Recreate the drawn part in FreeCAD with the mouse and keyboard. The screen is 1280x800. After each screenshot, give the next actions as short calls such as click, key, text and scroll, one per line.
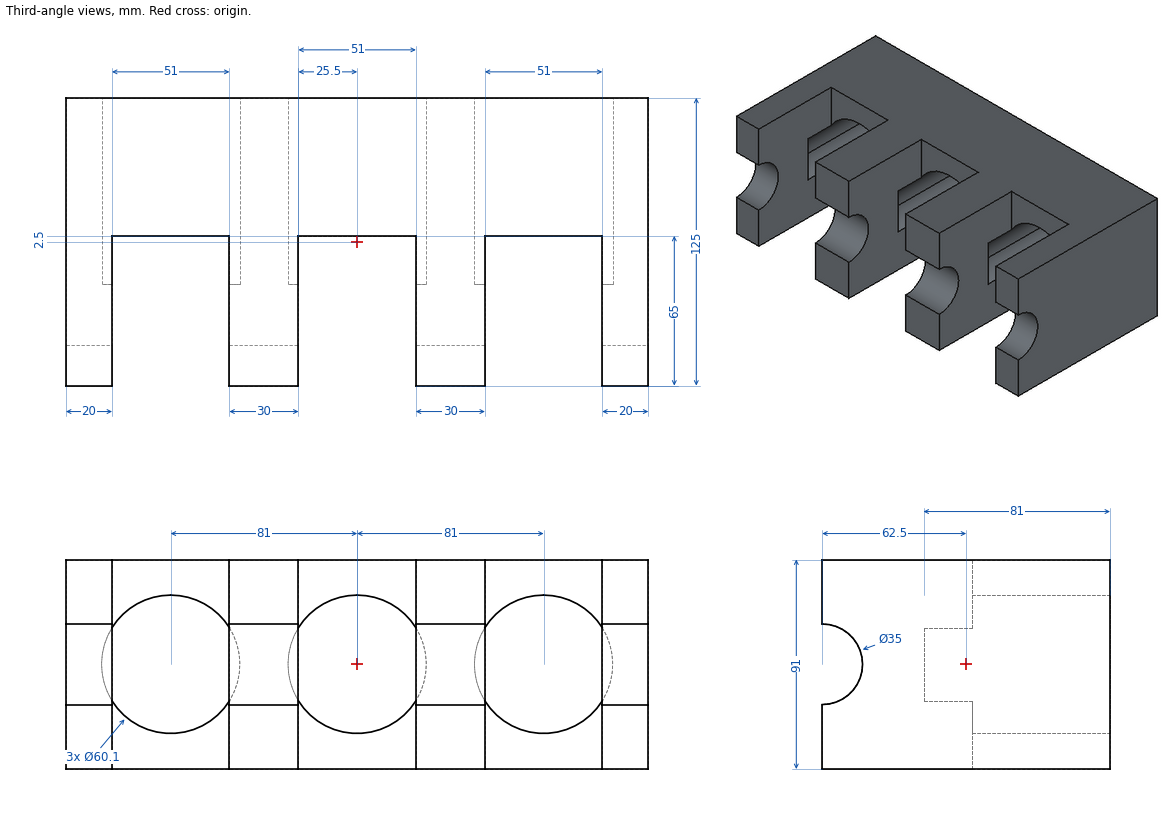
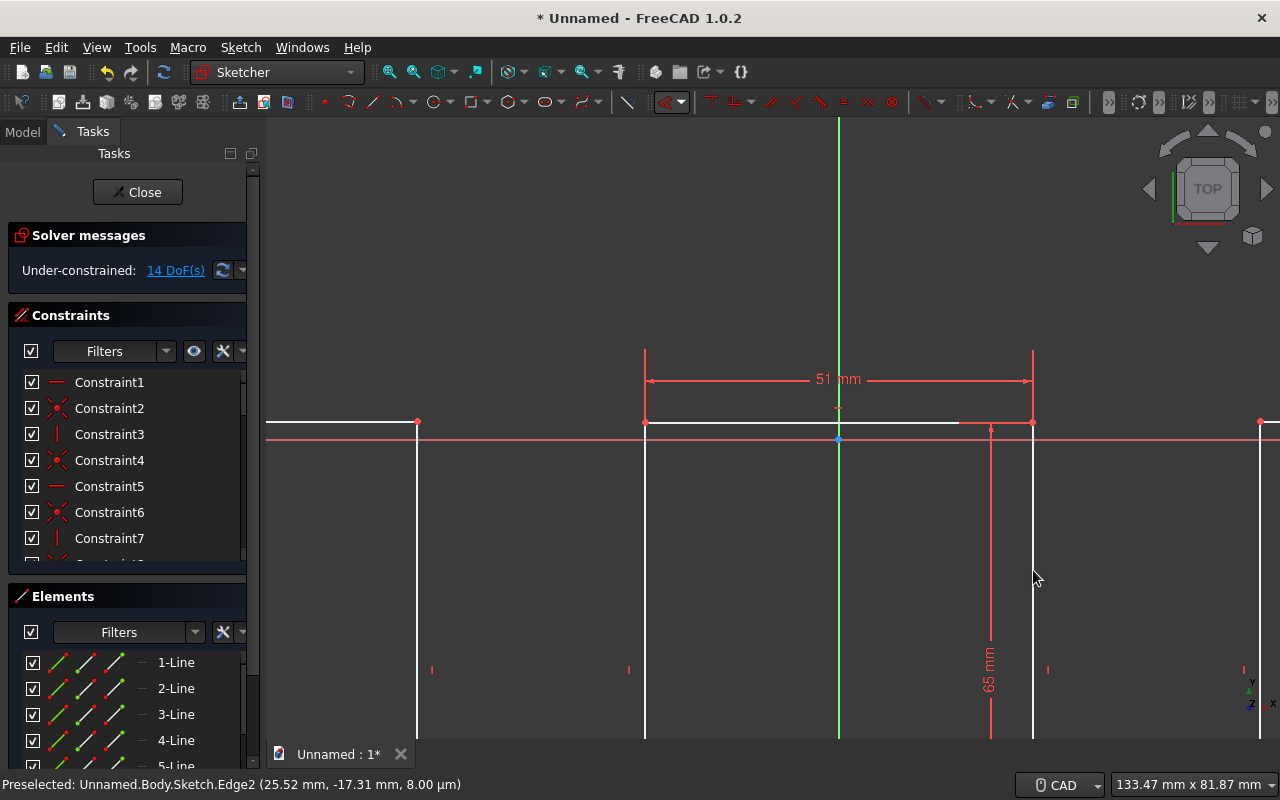
scroll(647, 423, down, 6)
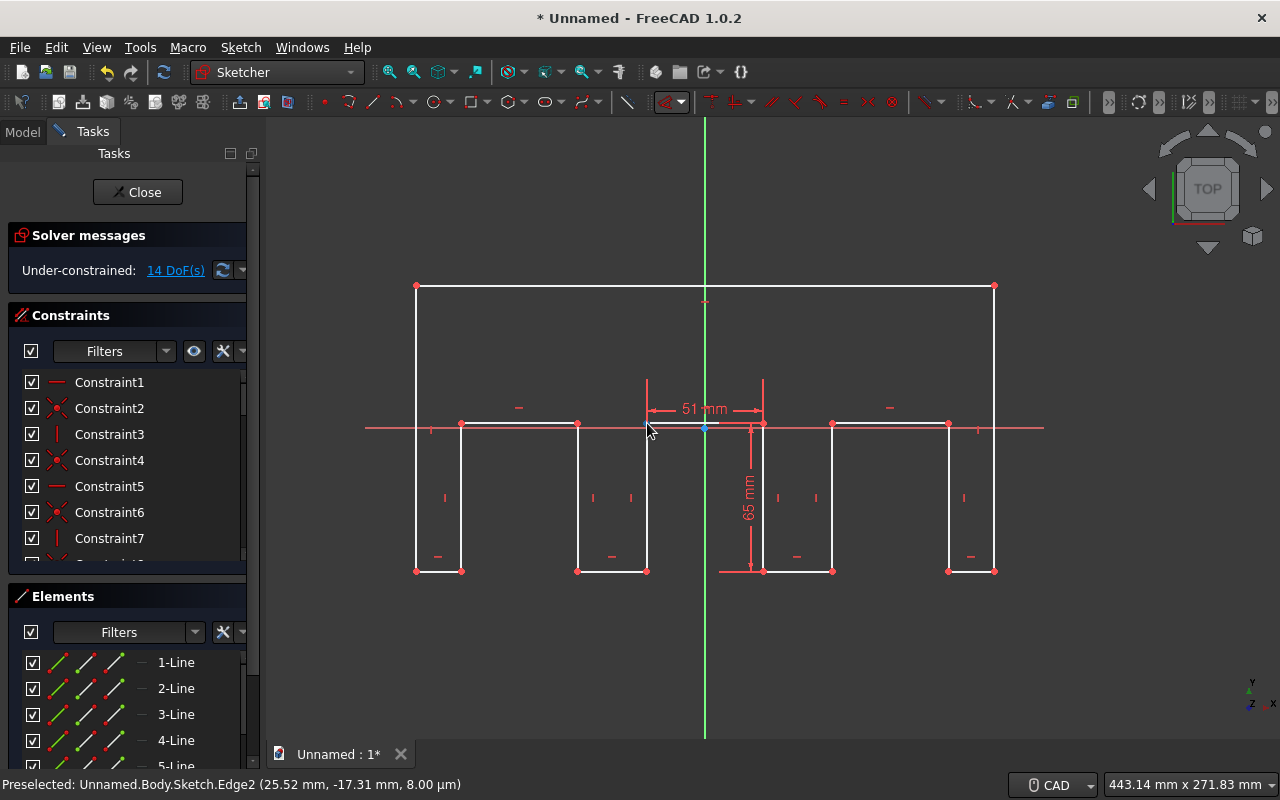
click(784, 572)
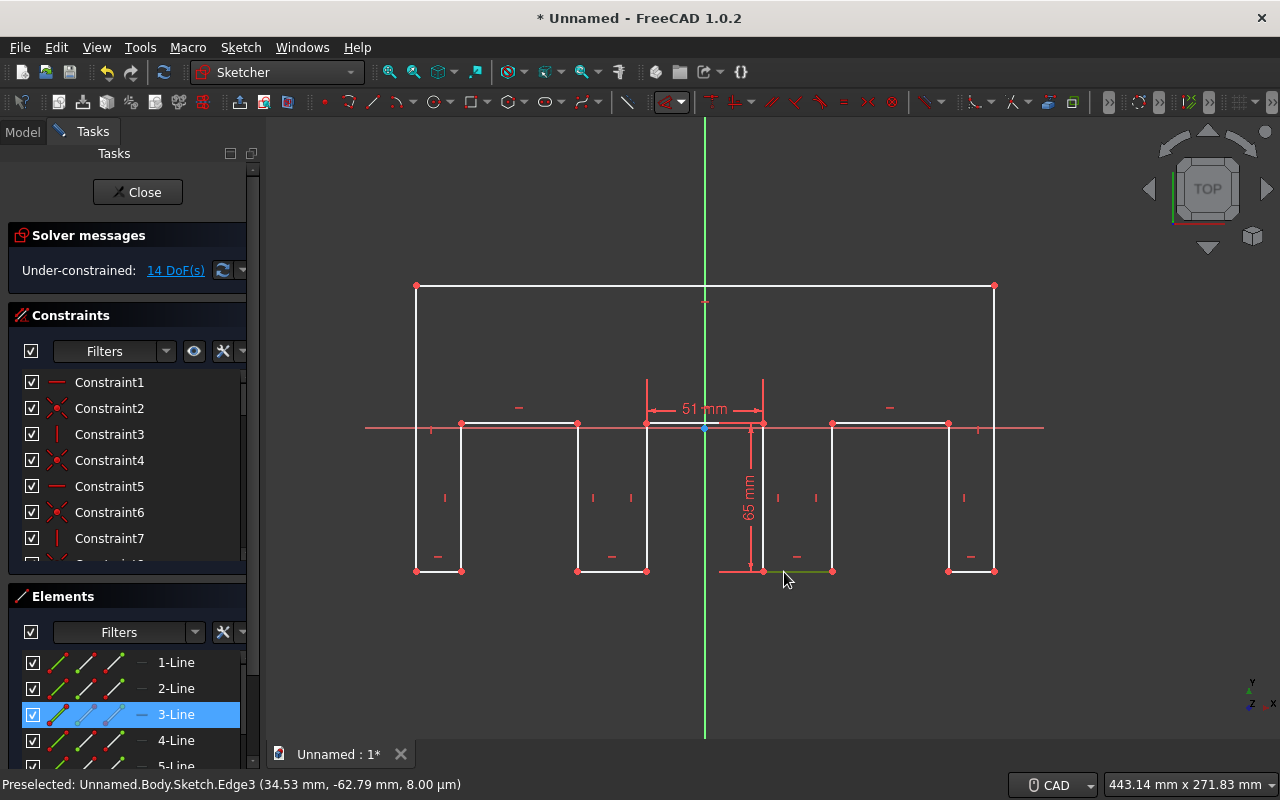
click(684, 102)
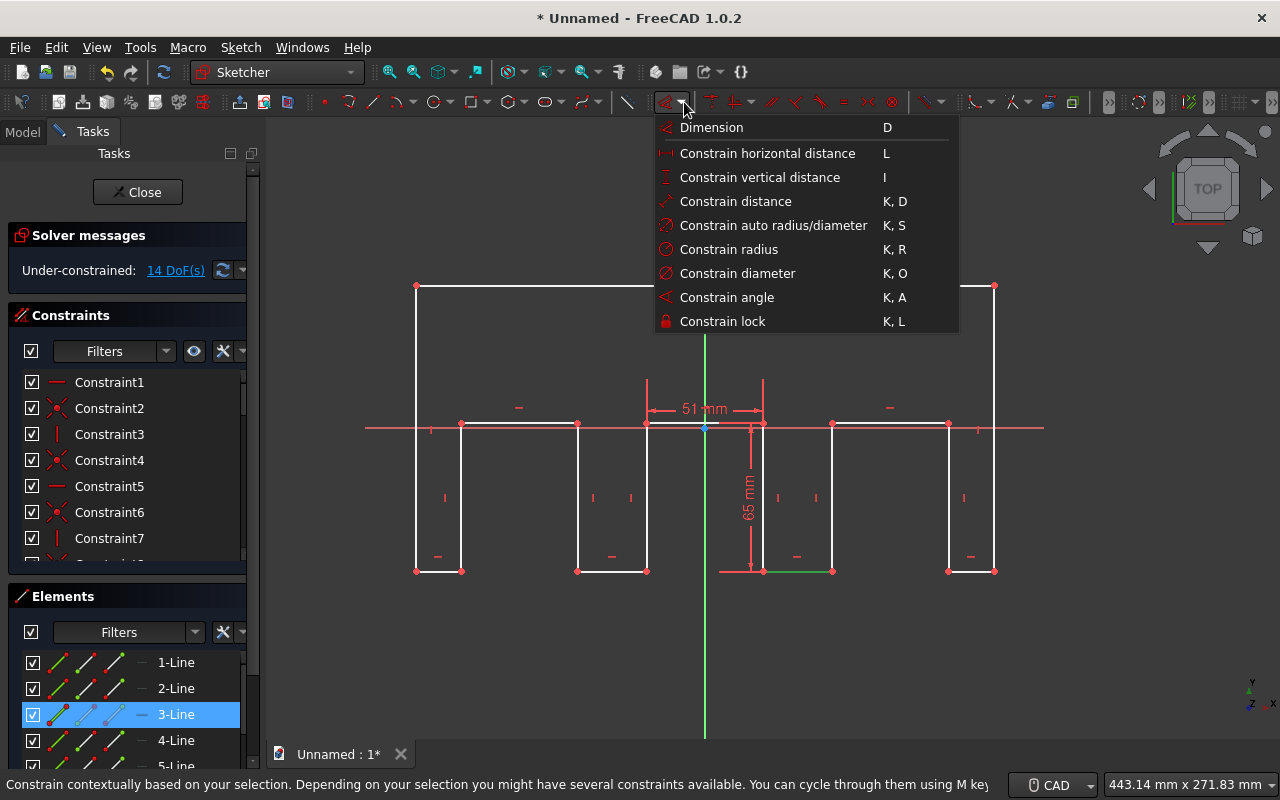
click(807, 153)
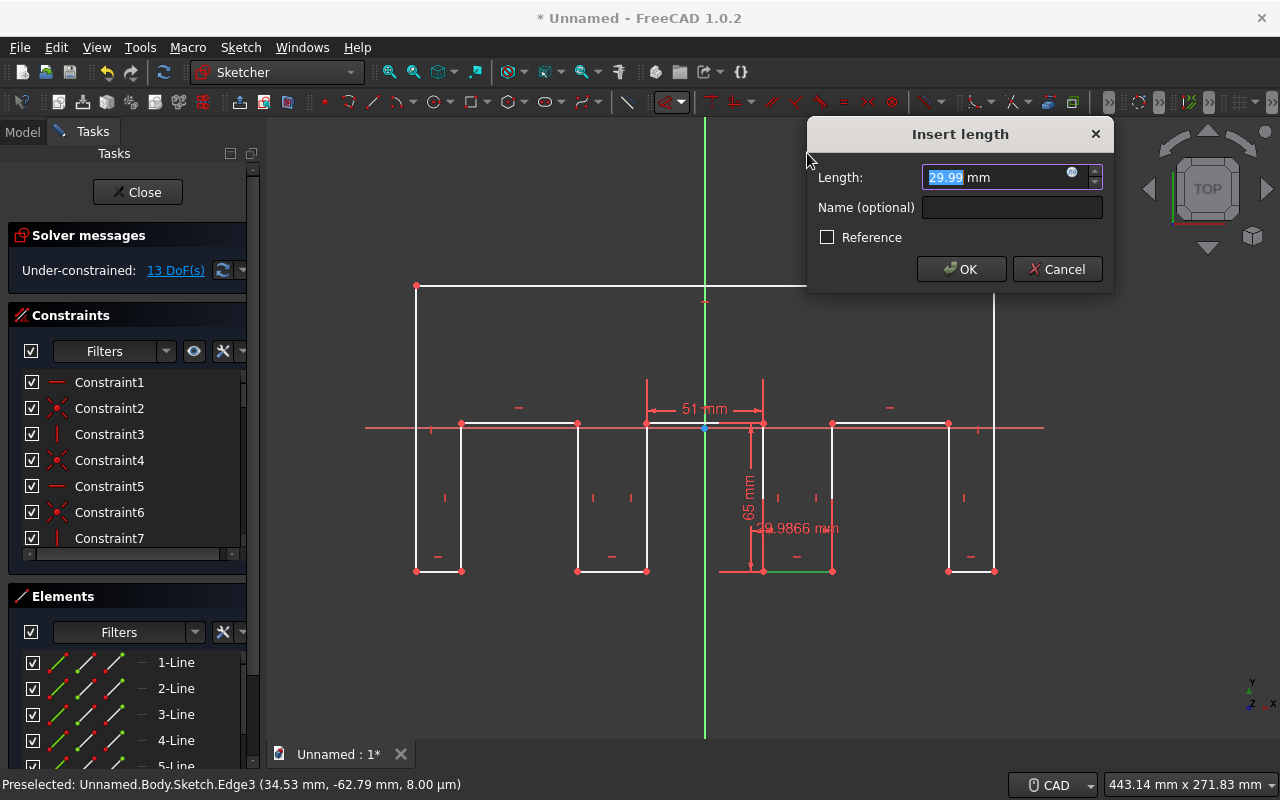
text(30)
key(Return)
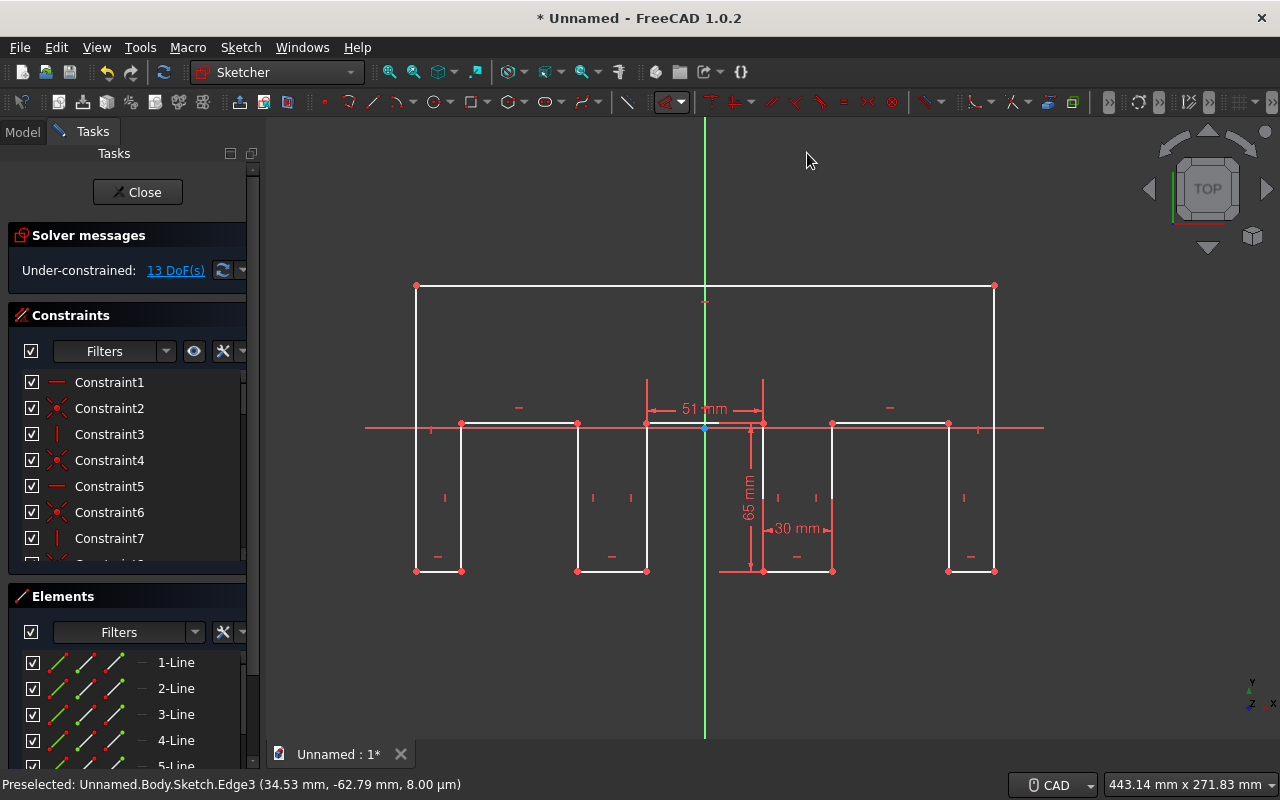
click(832, 527)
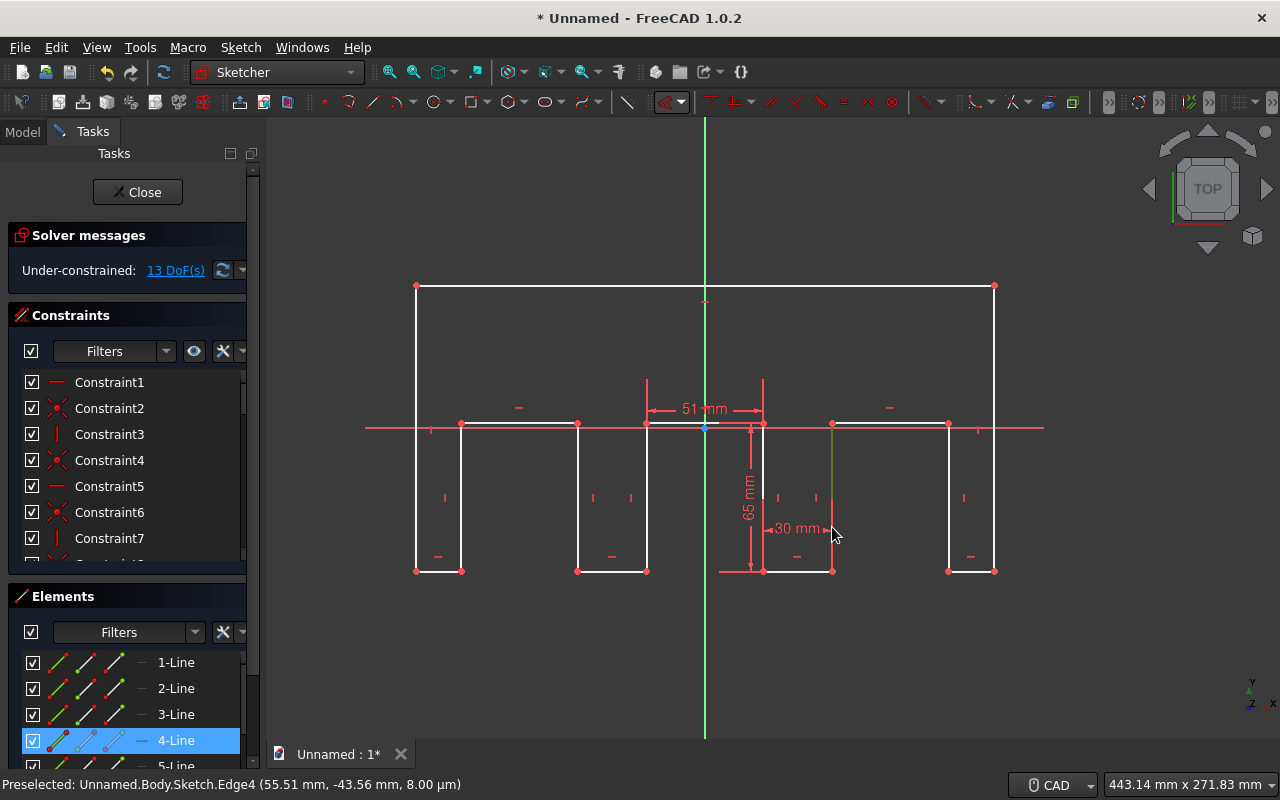
key(i)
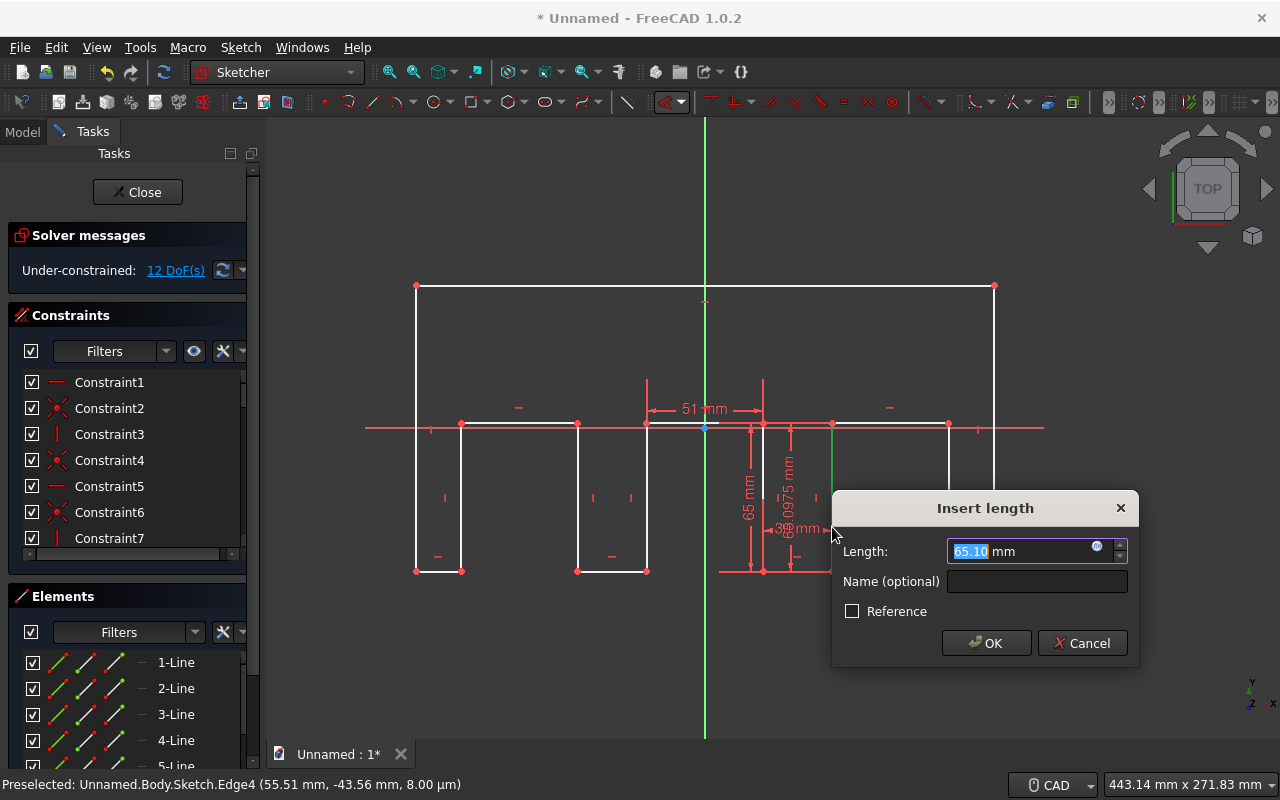
text(65)
key(Return)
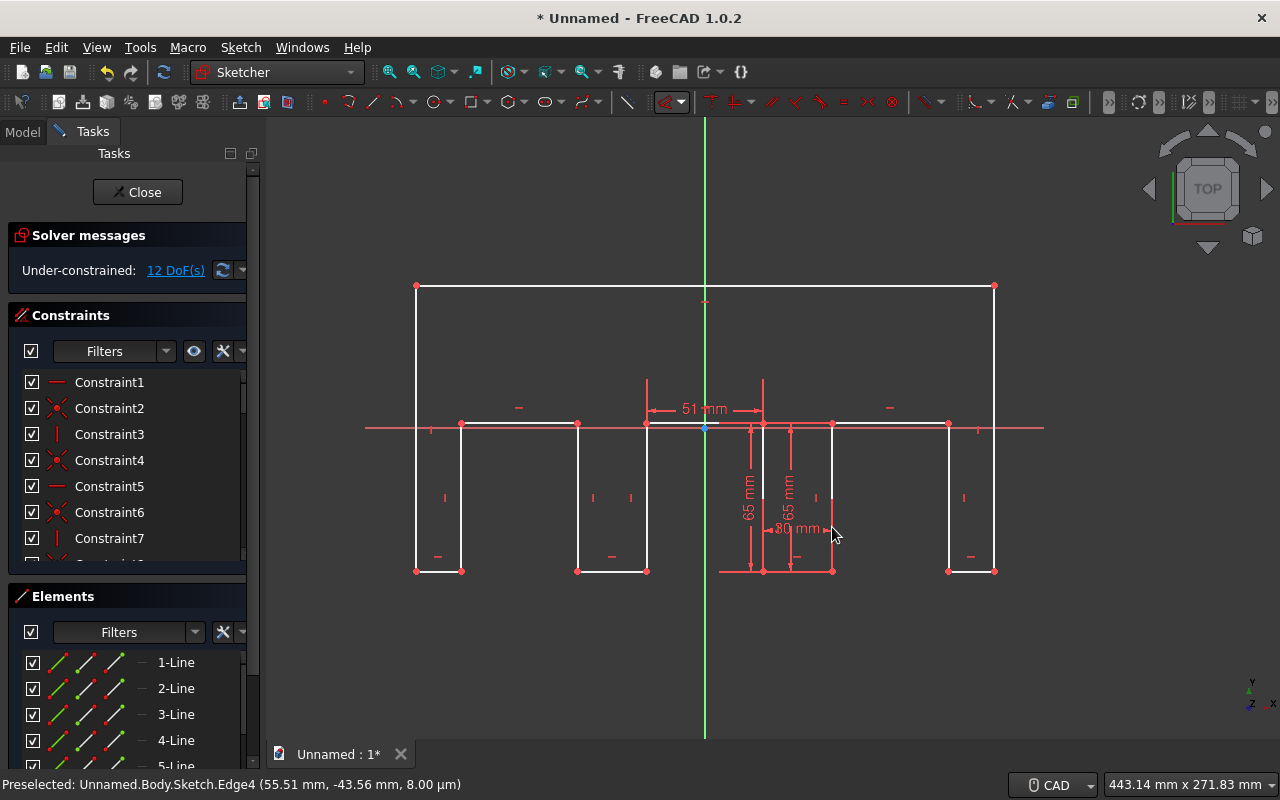
scroll(867, 423, up, 6)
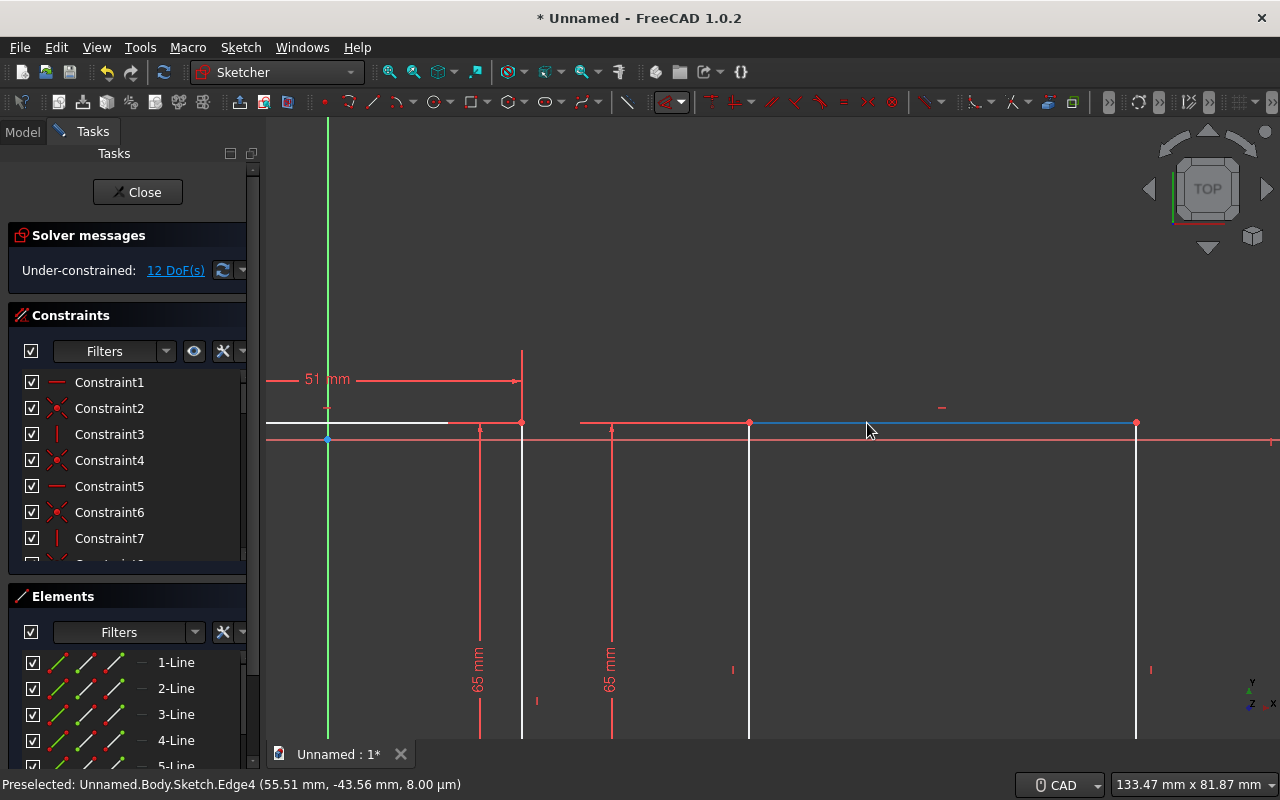
click(866, 423)